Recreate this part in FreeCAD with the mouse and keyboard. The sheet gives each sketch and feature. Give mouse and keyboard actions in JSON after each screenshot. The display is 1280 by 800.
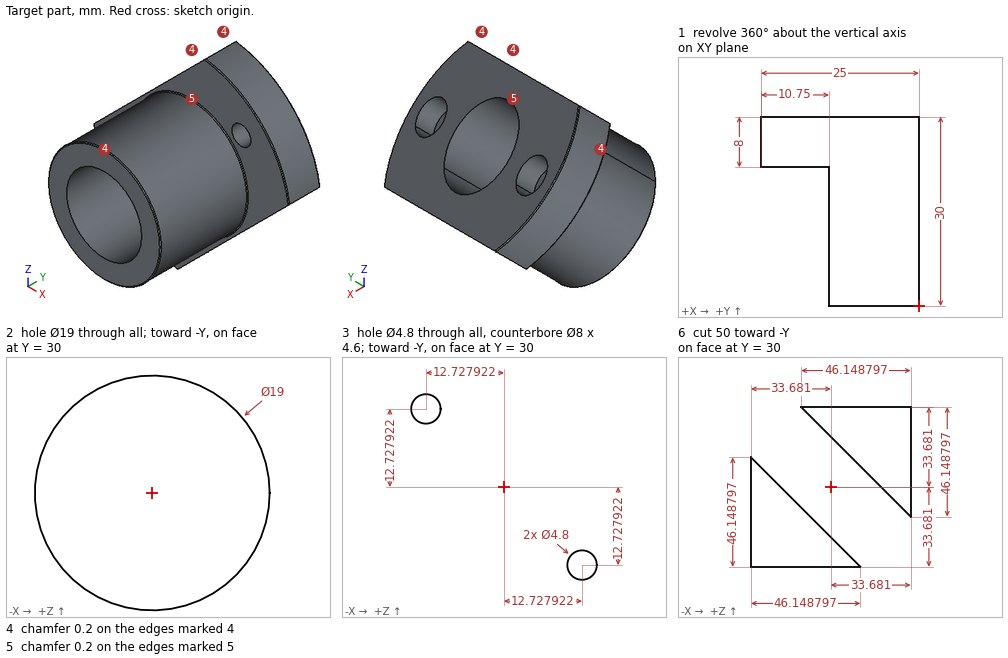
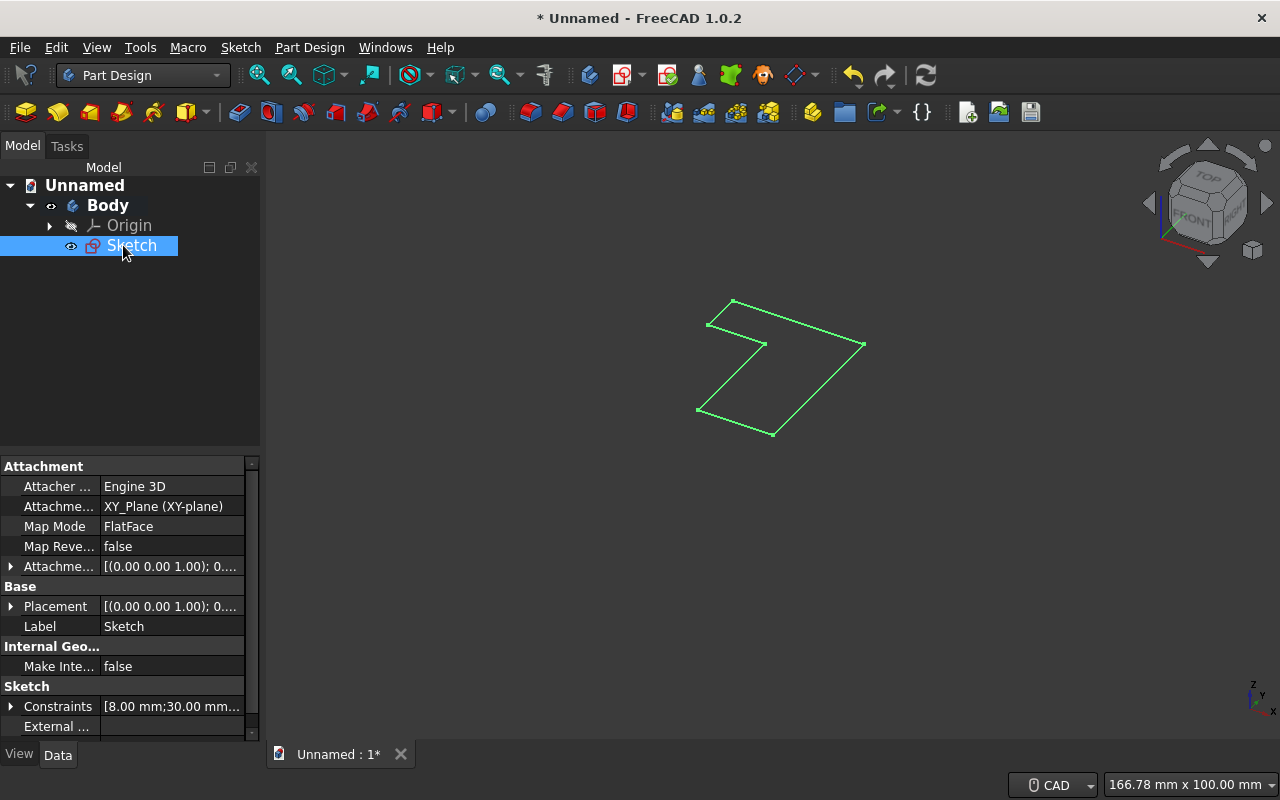
{"action": "left_click", "coordinate": [58, 112]}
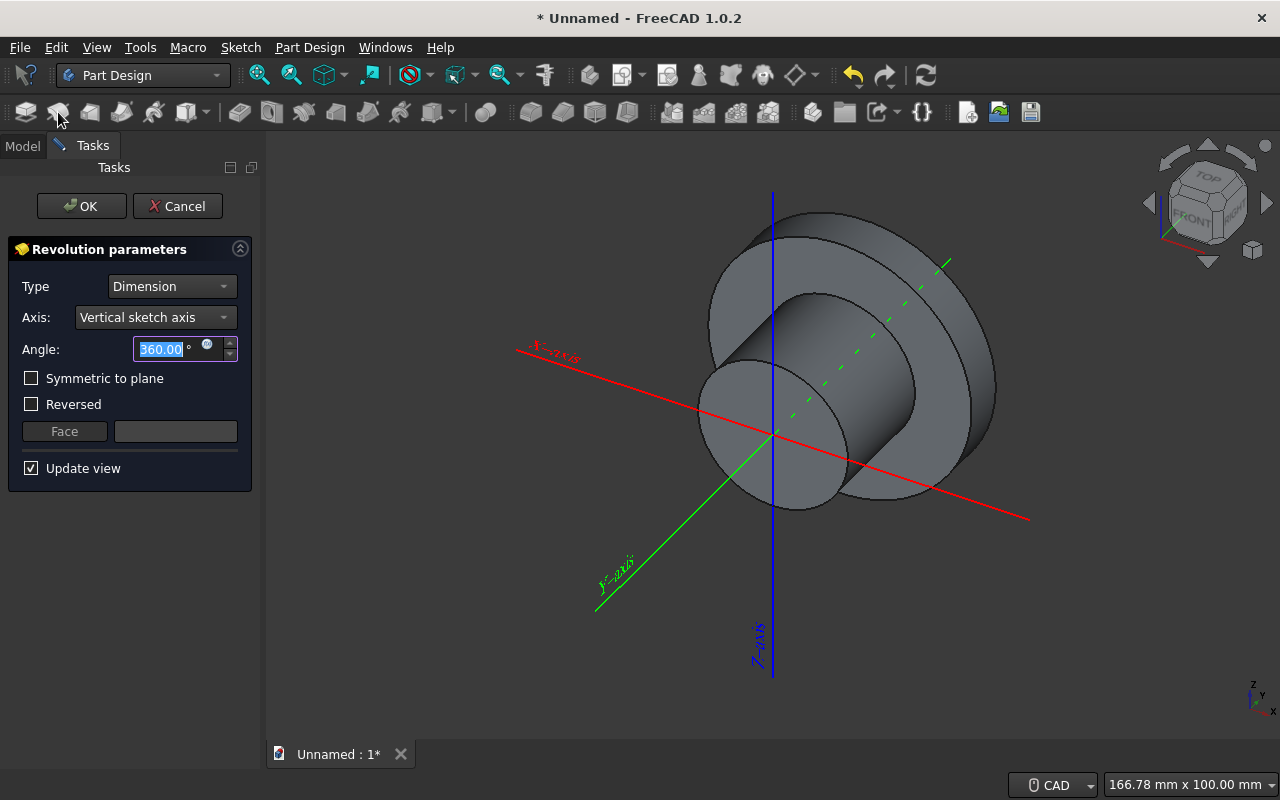
{"action": "left_click", "coordinate": [82, 206]}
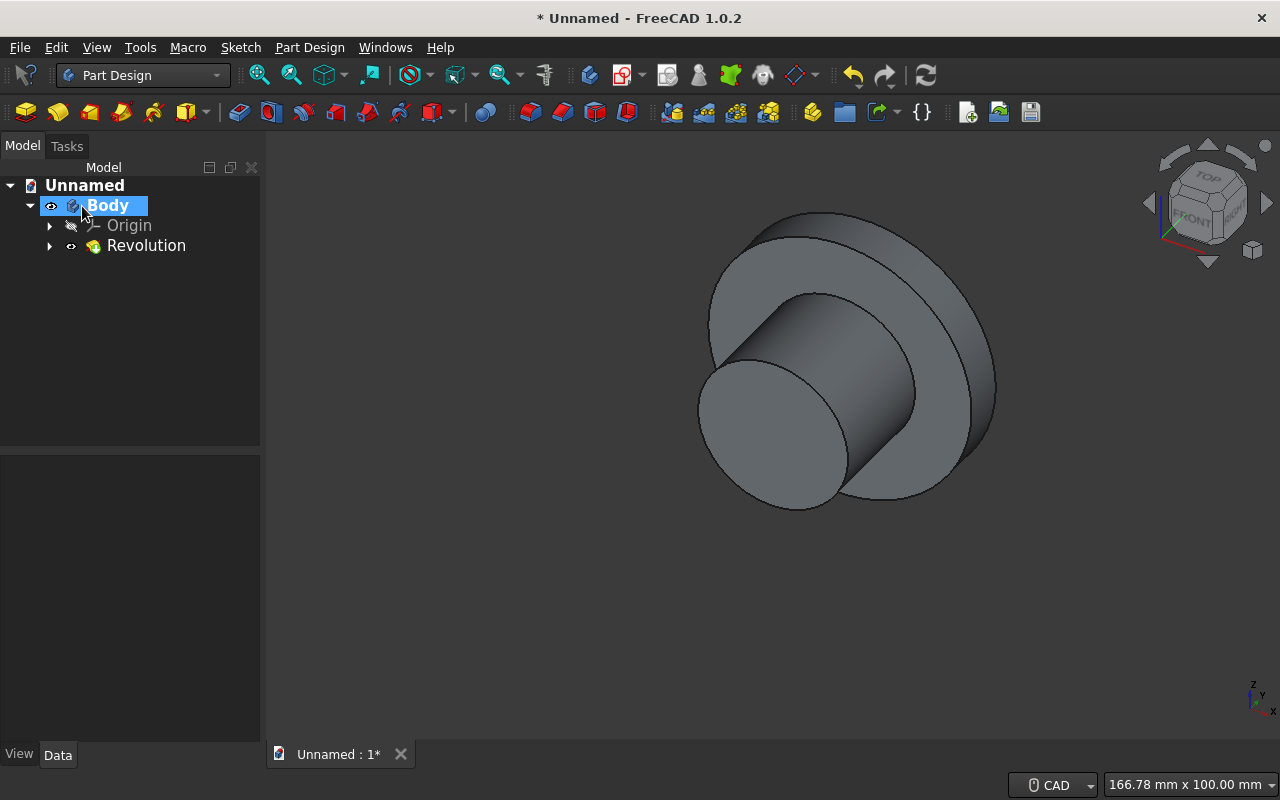
{"action": "key", "text": "4"}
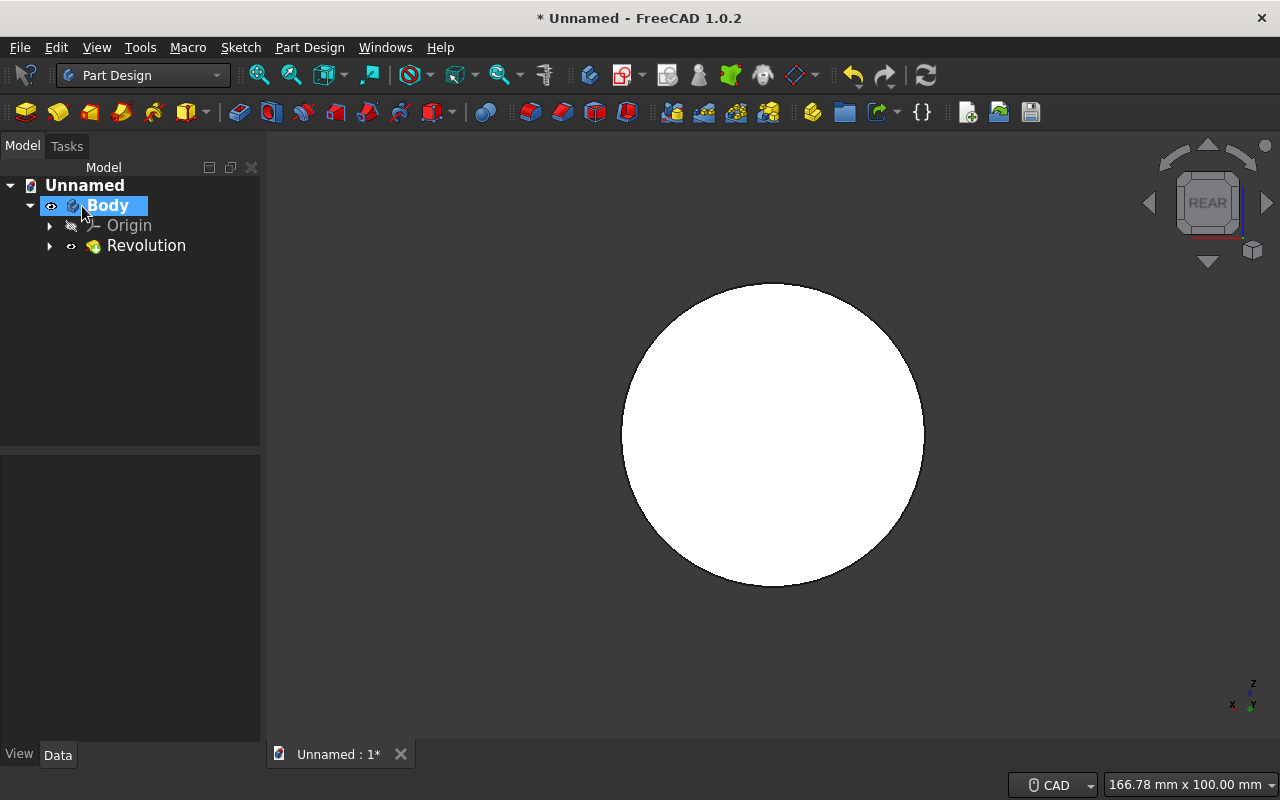
{"action": "left_click", "coordinate": [773, 434]}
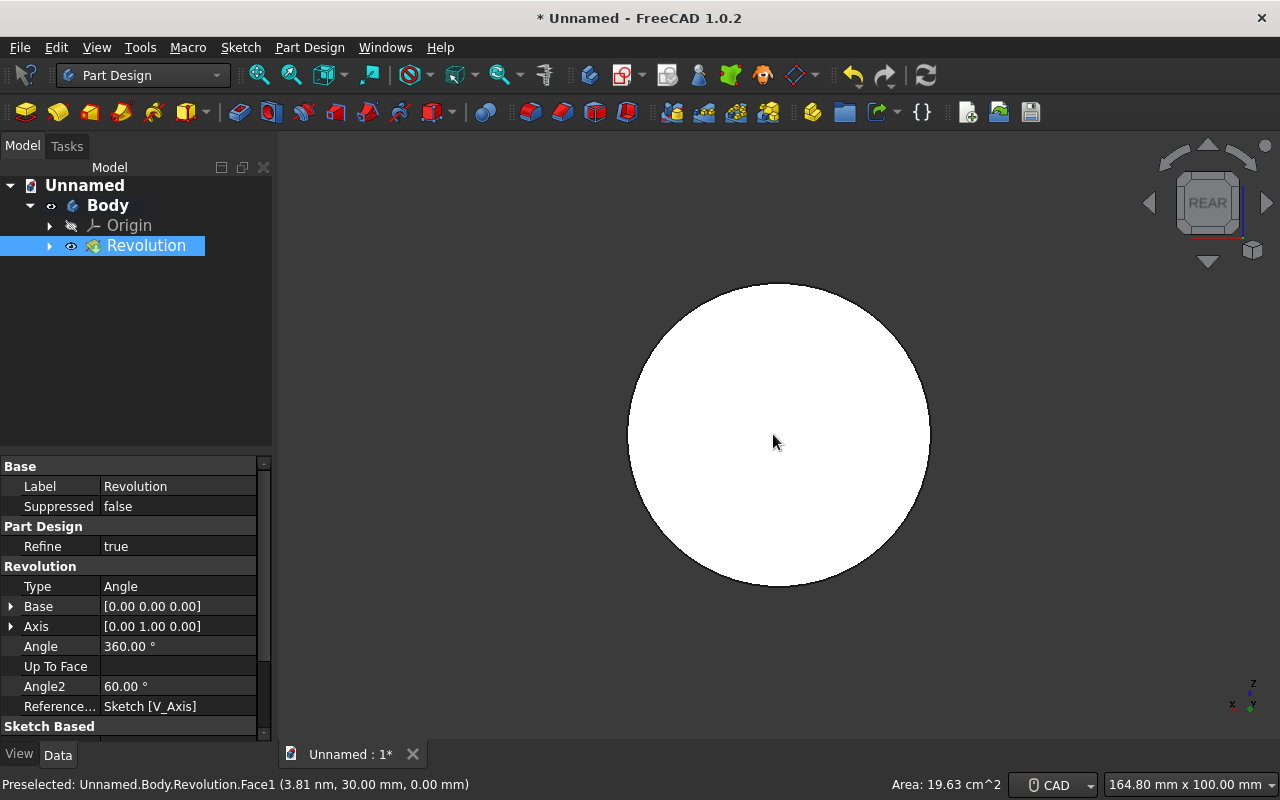
{"action": "left_click", "coordinate": [622, 76]}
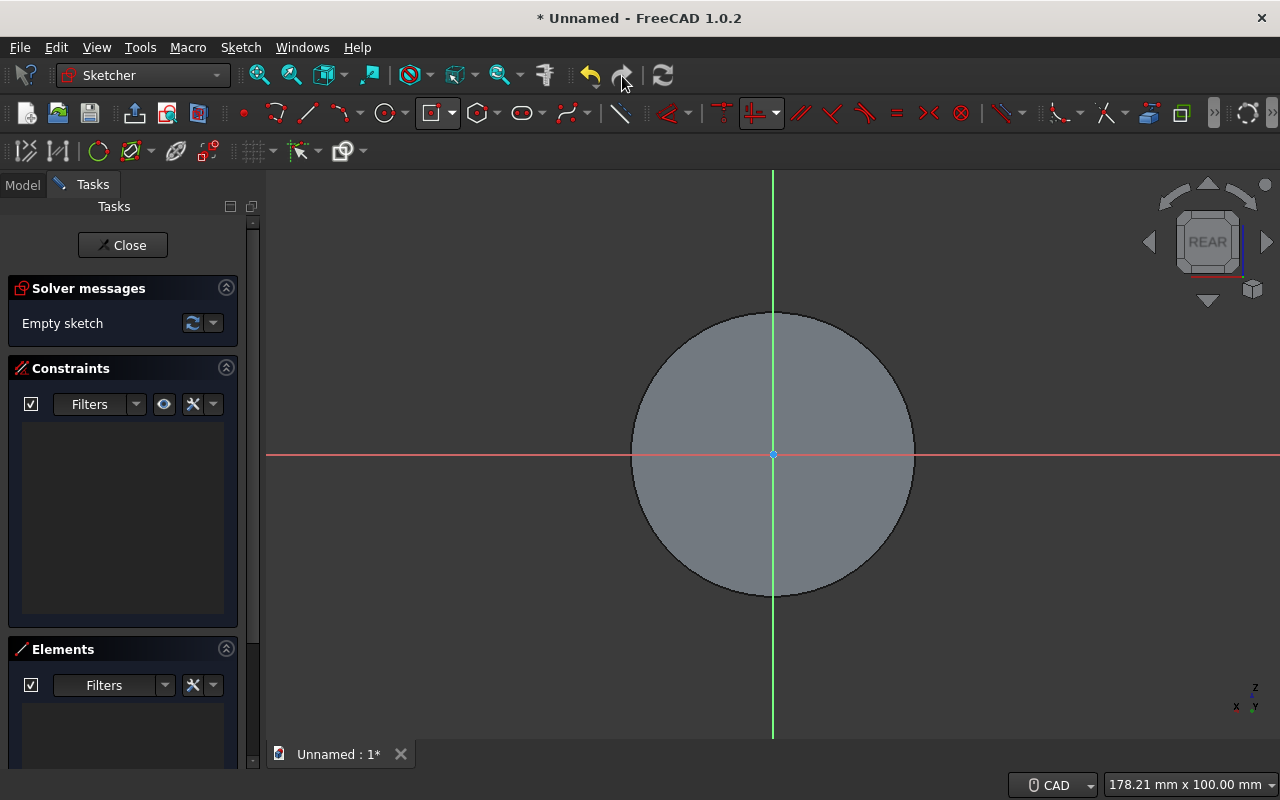
{"action": "scroll", "coordinate": [803, 454], "scroll_direction": "up", "scroll_amount": 6}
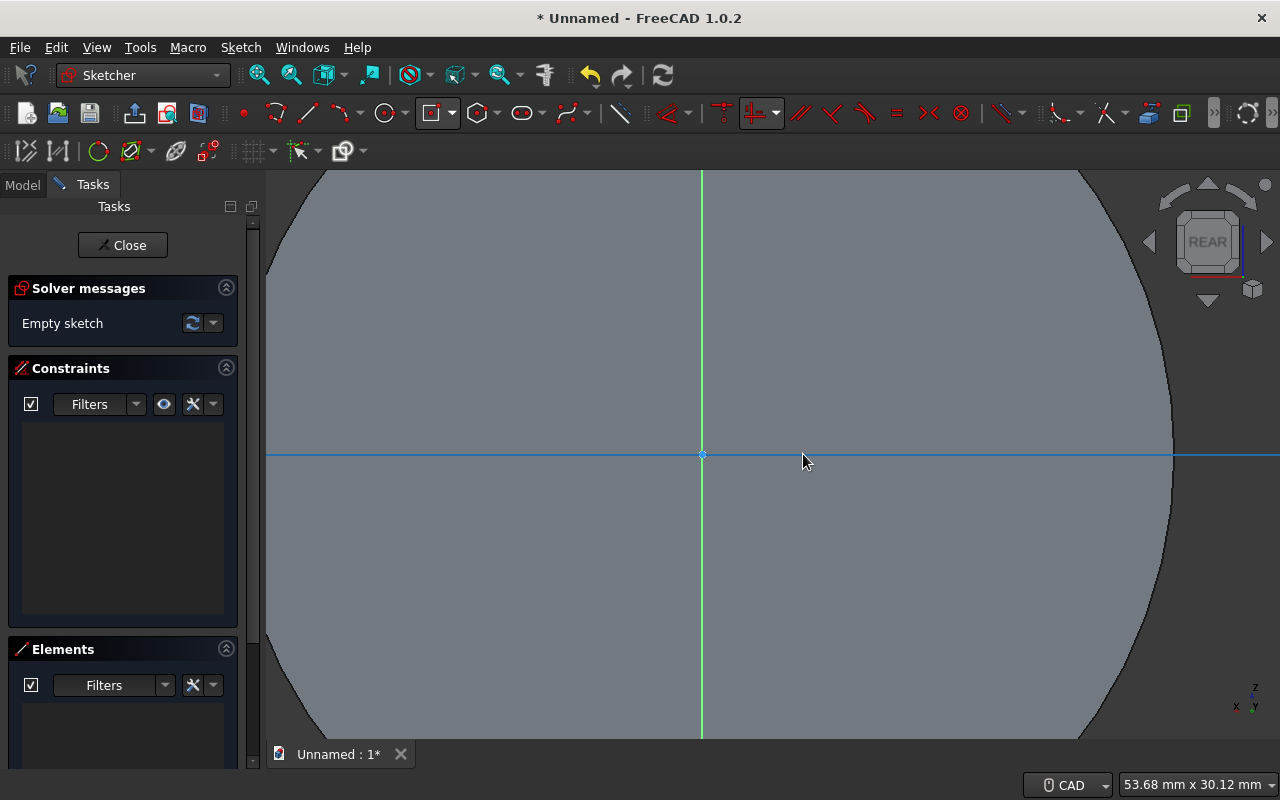
{"action": "left_click", "coordinate": [386, 114]}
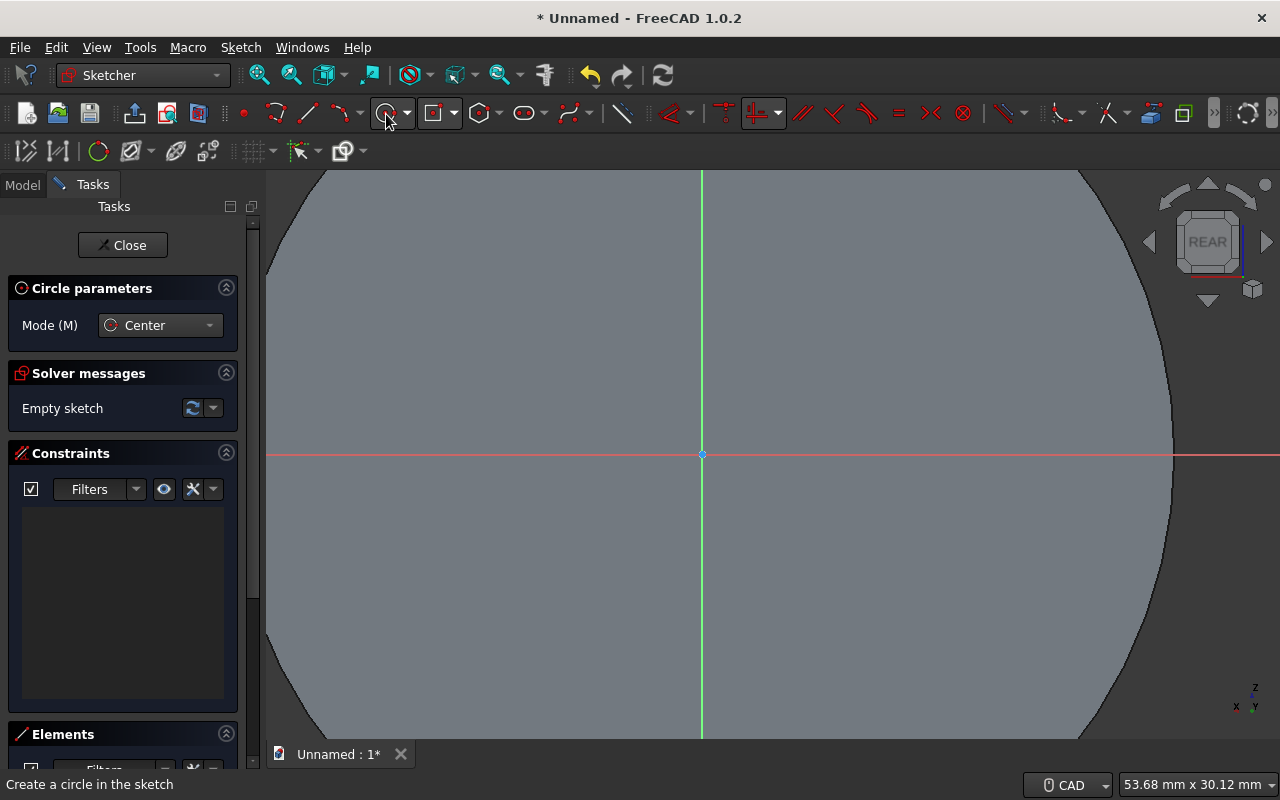
{"action": "left_click", "coordinate": [702, 454]}
{"action": "mouse_move", "coordinate": [829, 328]}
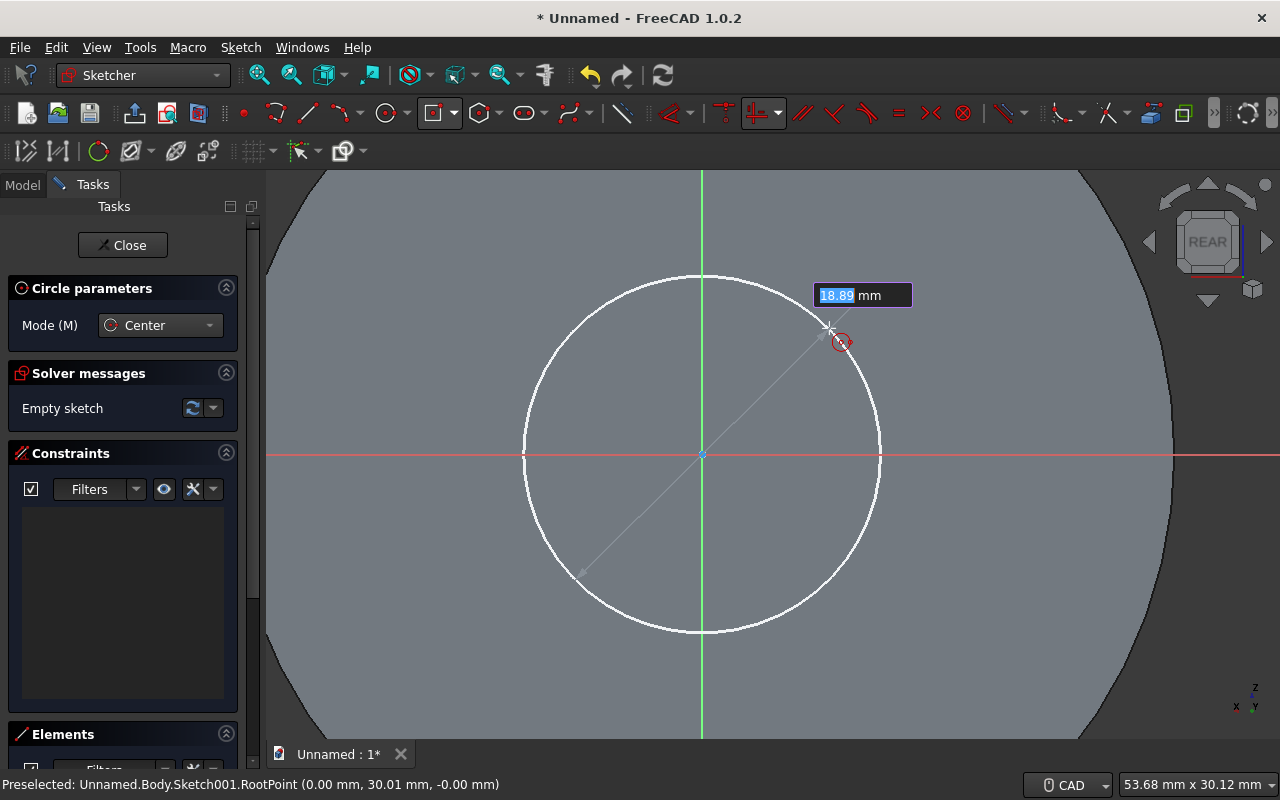
{"action": "type", "text": "19"}
{"action": "key", "text": "Return"}
{"action": "key", "text": "Escape"}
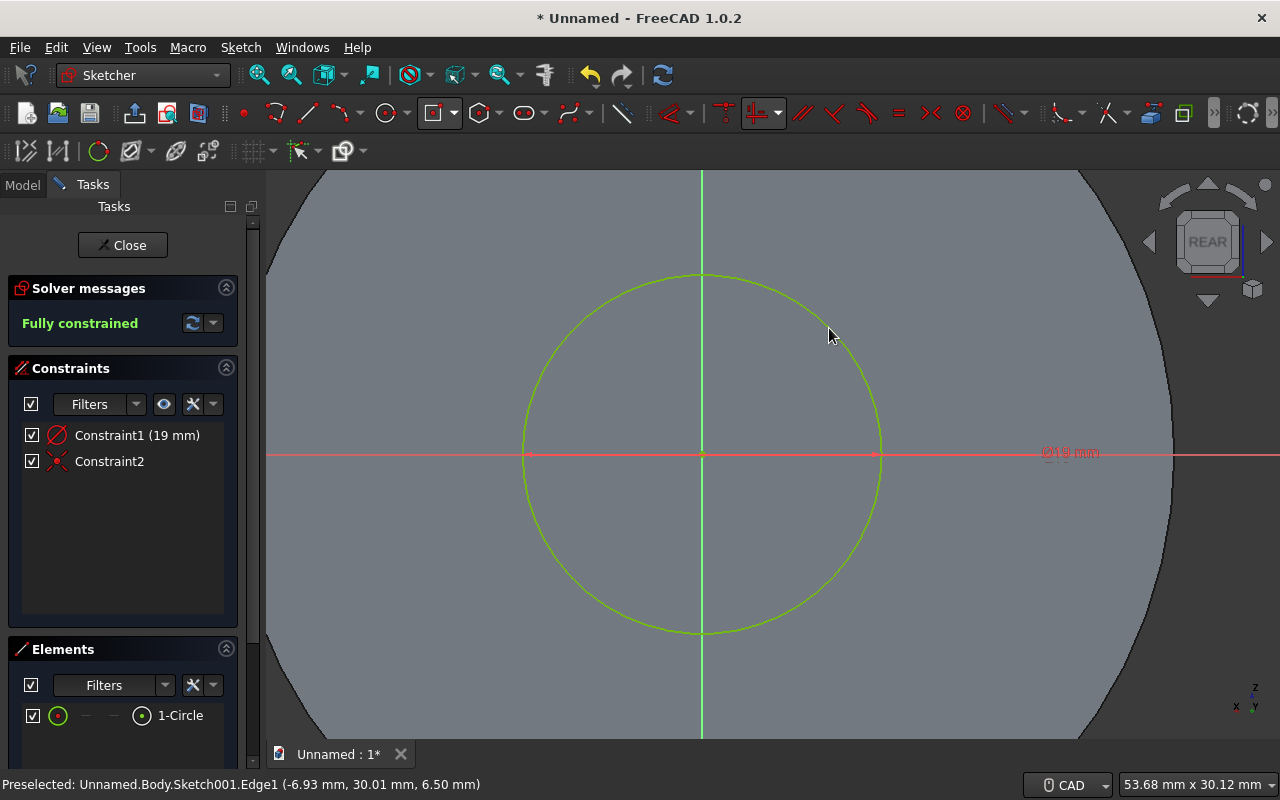
{"action": "left_click", "coordinate": [123, 245]}